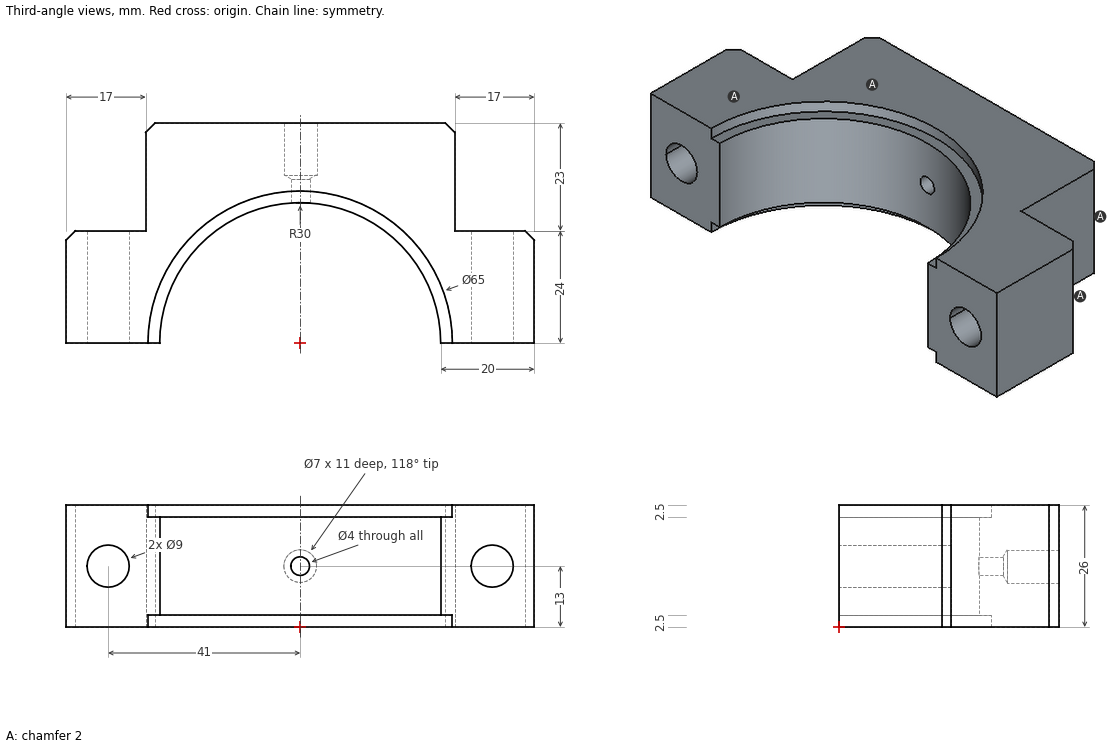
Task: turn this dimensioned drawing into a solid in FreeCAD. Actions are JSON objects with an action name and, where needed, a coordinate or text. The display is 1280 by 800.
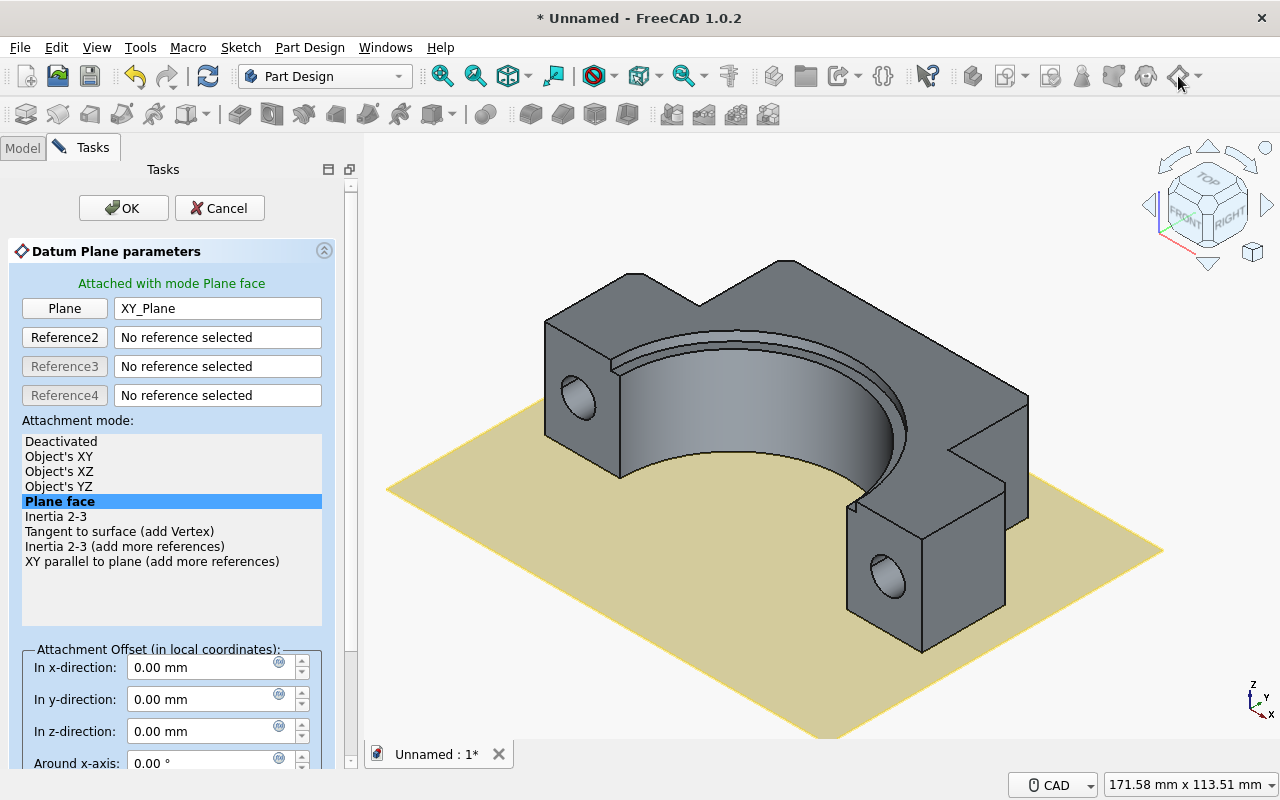
{"action": "triple_click", "coordinate": [210, 731]}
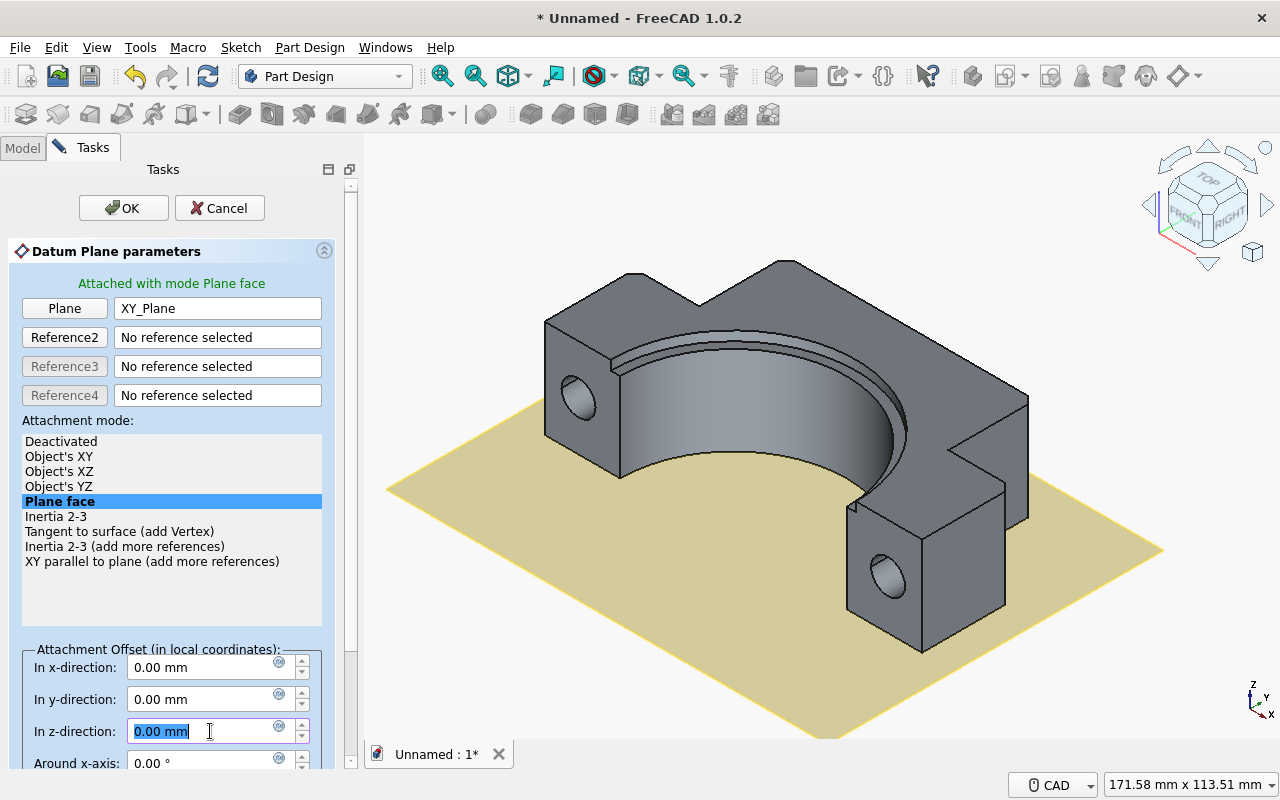
{"action": "type", "text": "2.5"}
{"action": "key", "text": "Tab"}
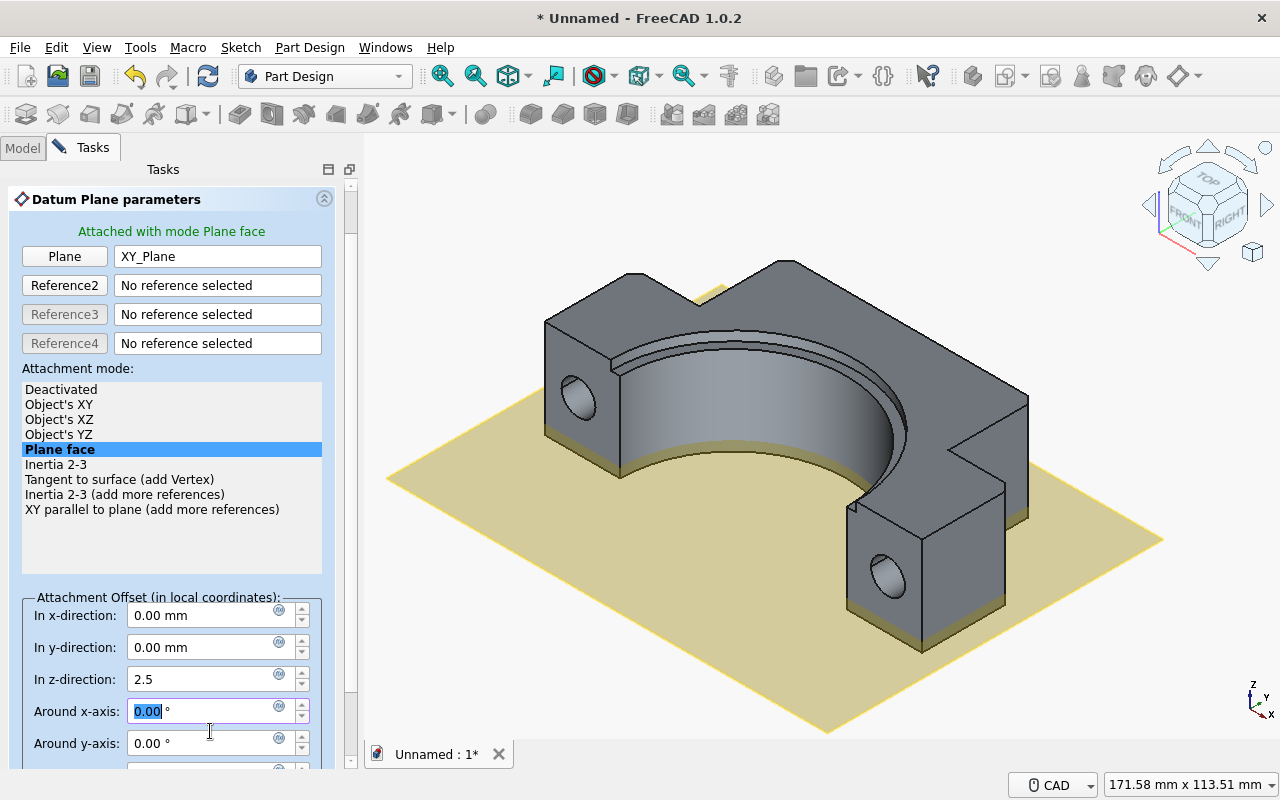
{"action": "scroll", "coordinate": [351, 474], "scroll_direction": "up", "scroll_amount": 2}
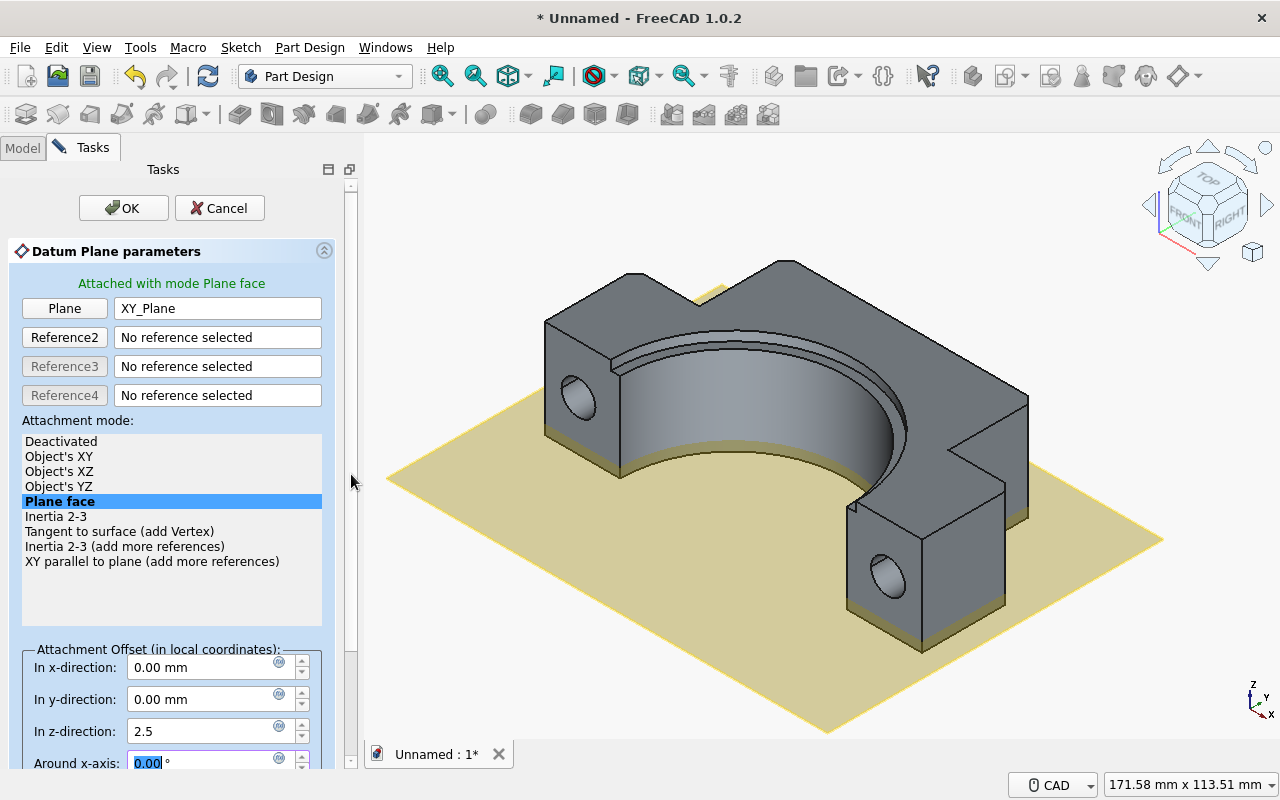
{"action": "left_click", "coordinate": [124, 208]}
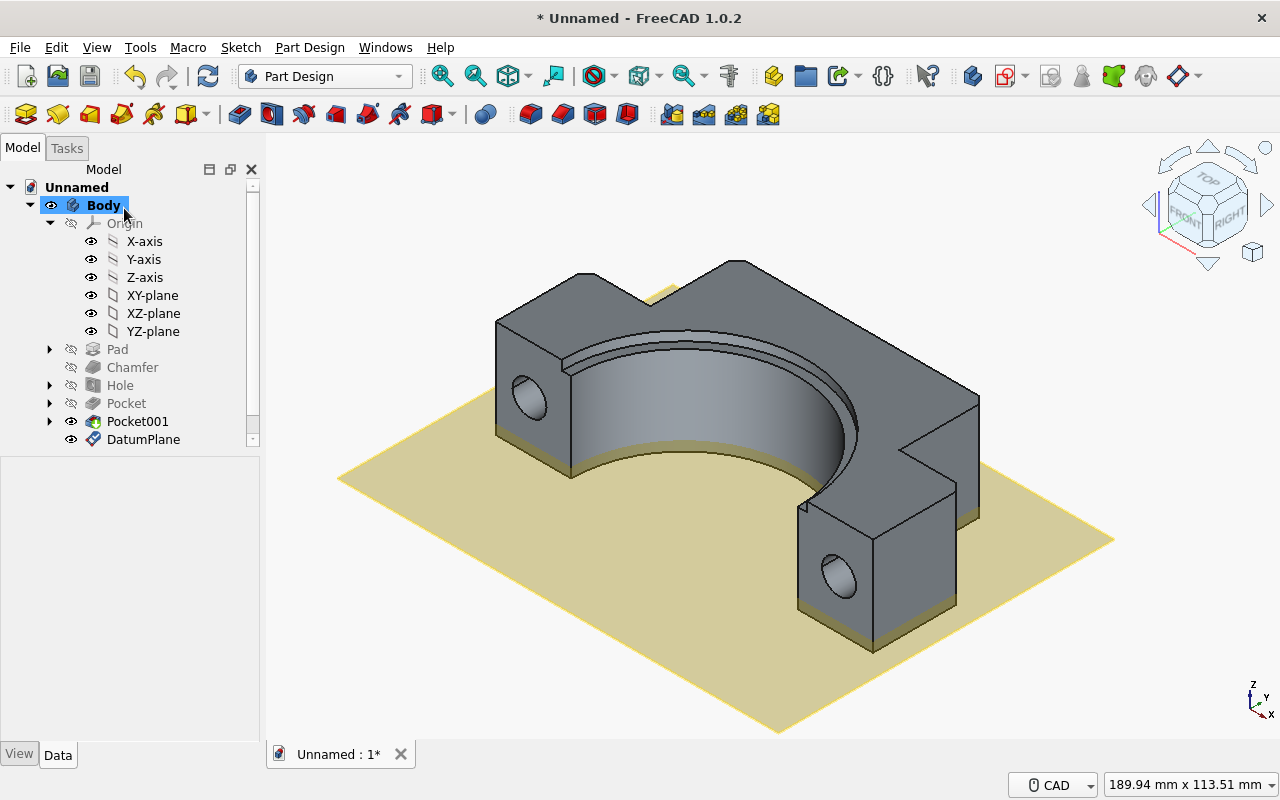
{"action": "left_click", "coordinate": [116, 439]}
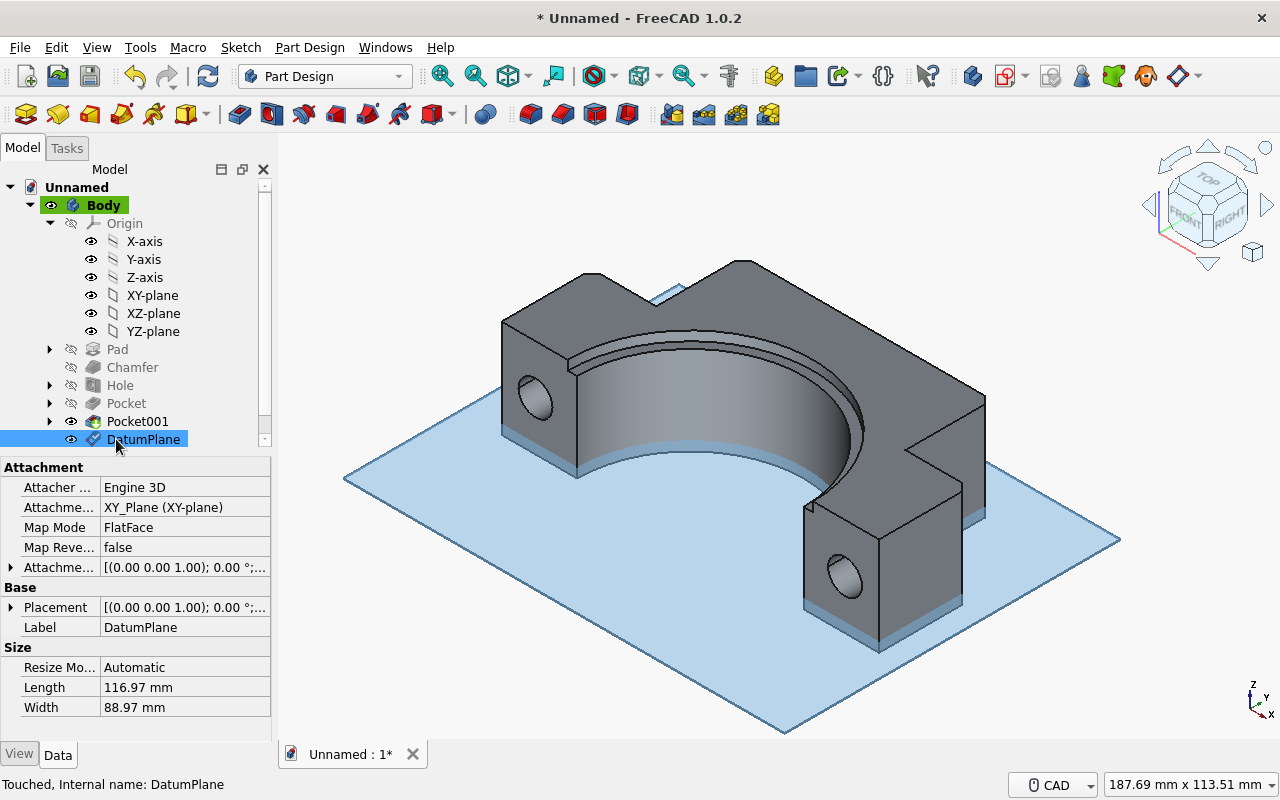
{"action": "left_click", "coordinate": [1006, 76]}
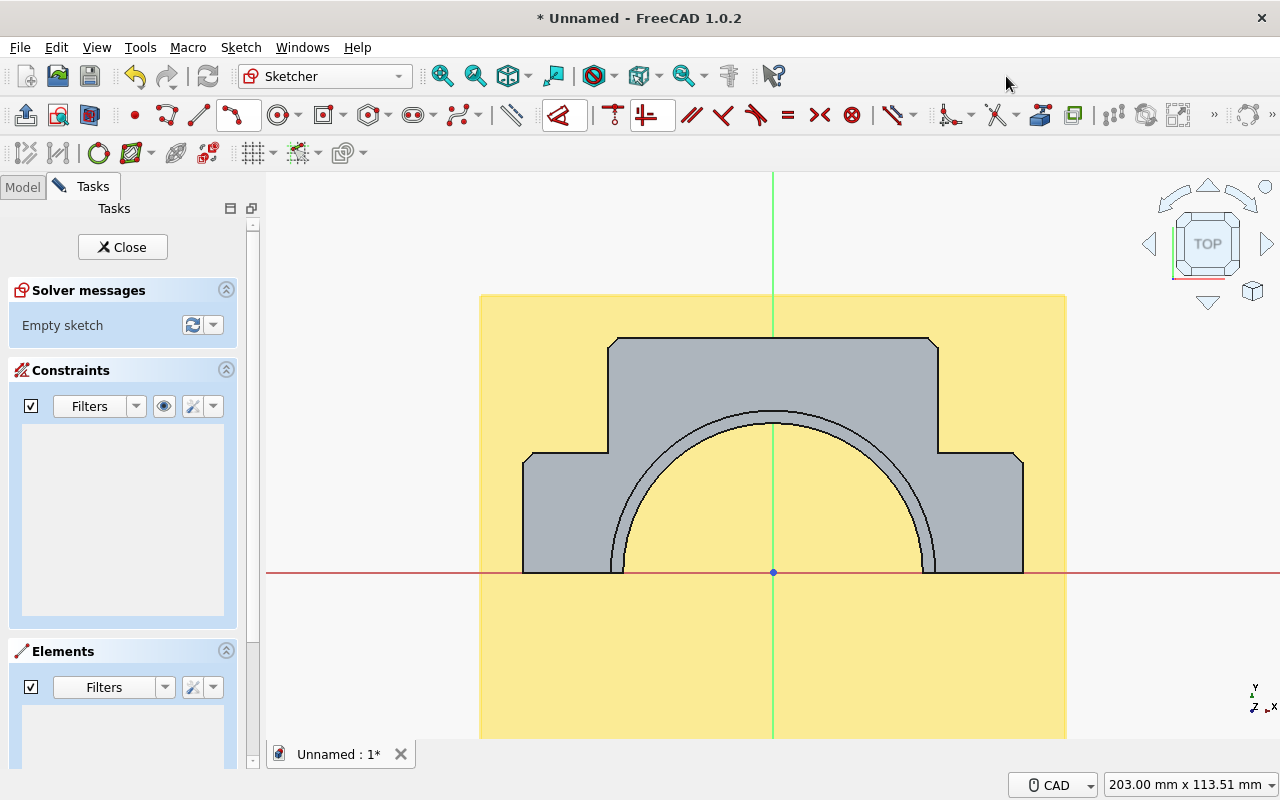
{"action": "key", "text": "q s"}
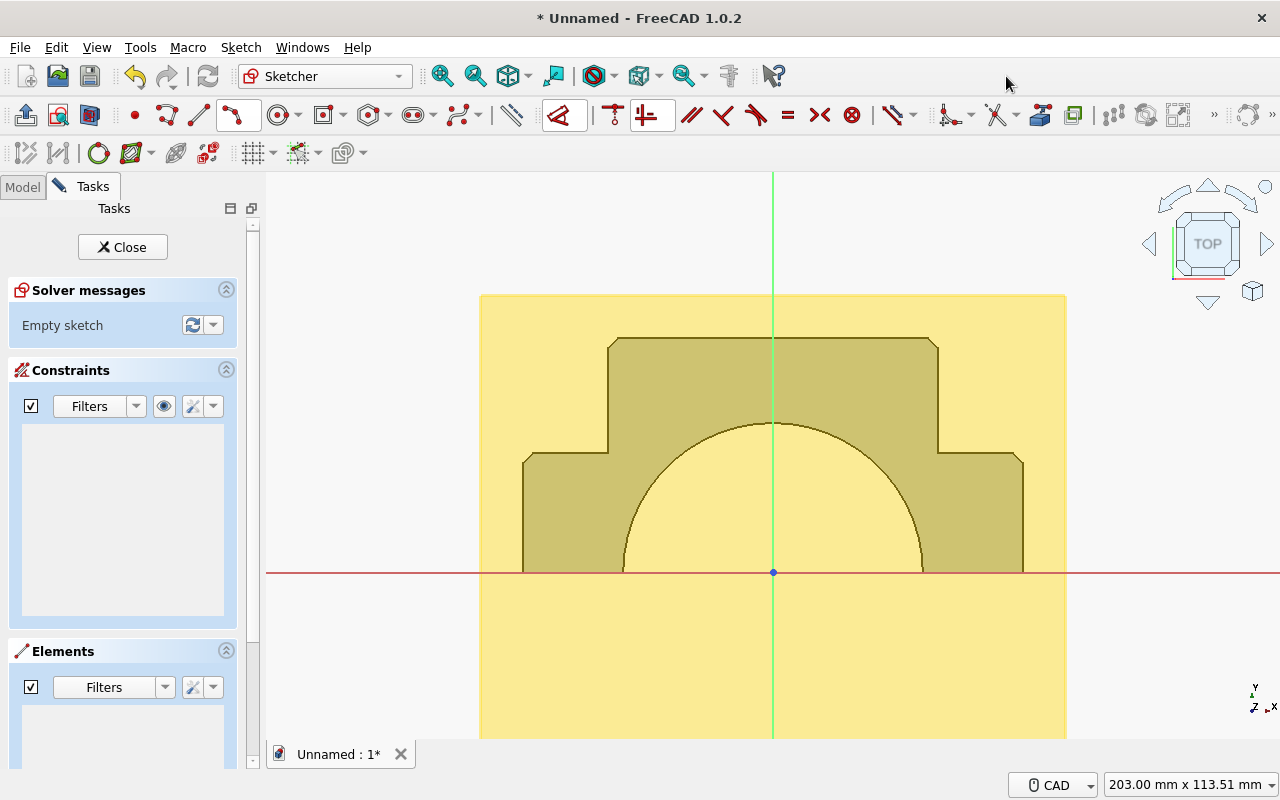
{"action": "scroll", "coordinate": [395, 200], "scroll_direction": "down", "scroll_amount": 1}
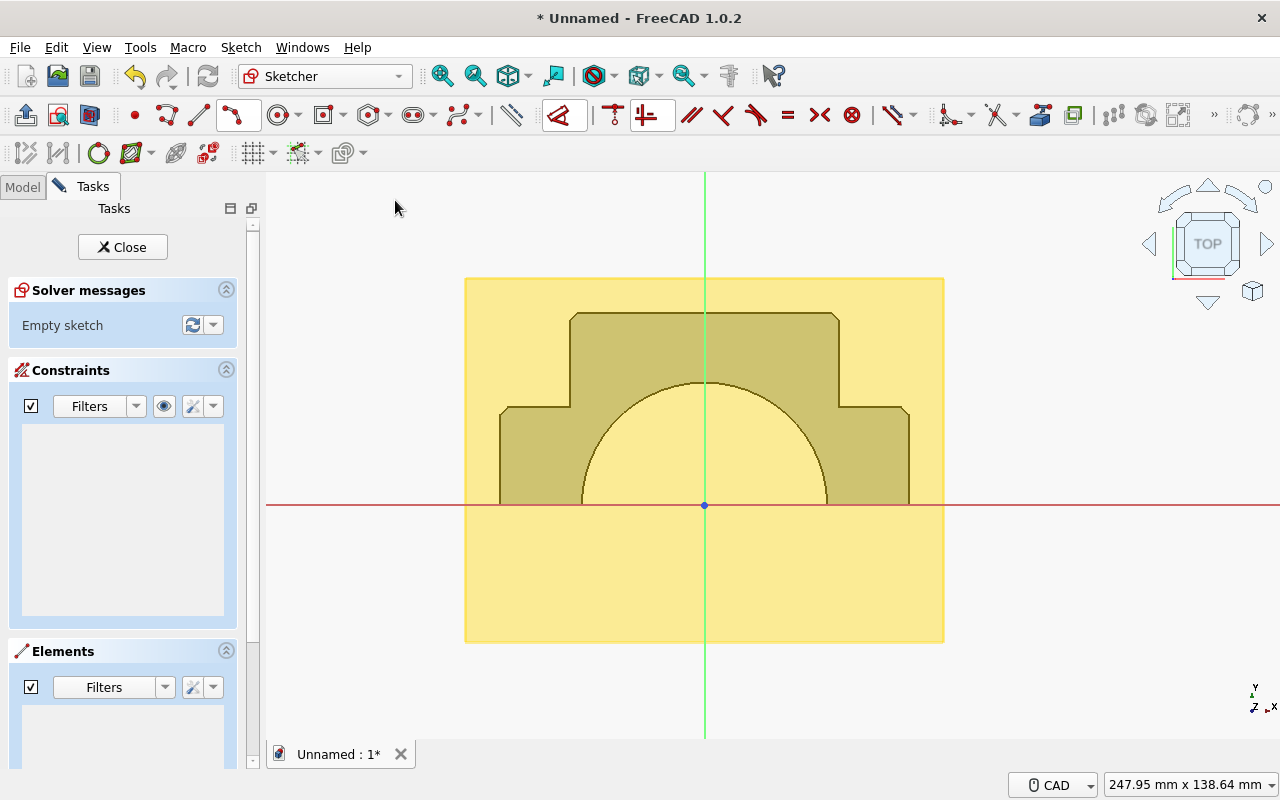
{"action": "scroll", "coordinate": [705, 607], "scroll_direction": "up", "scroll_amount": 2}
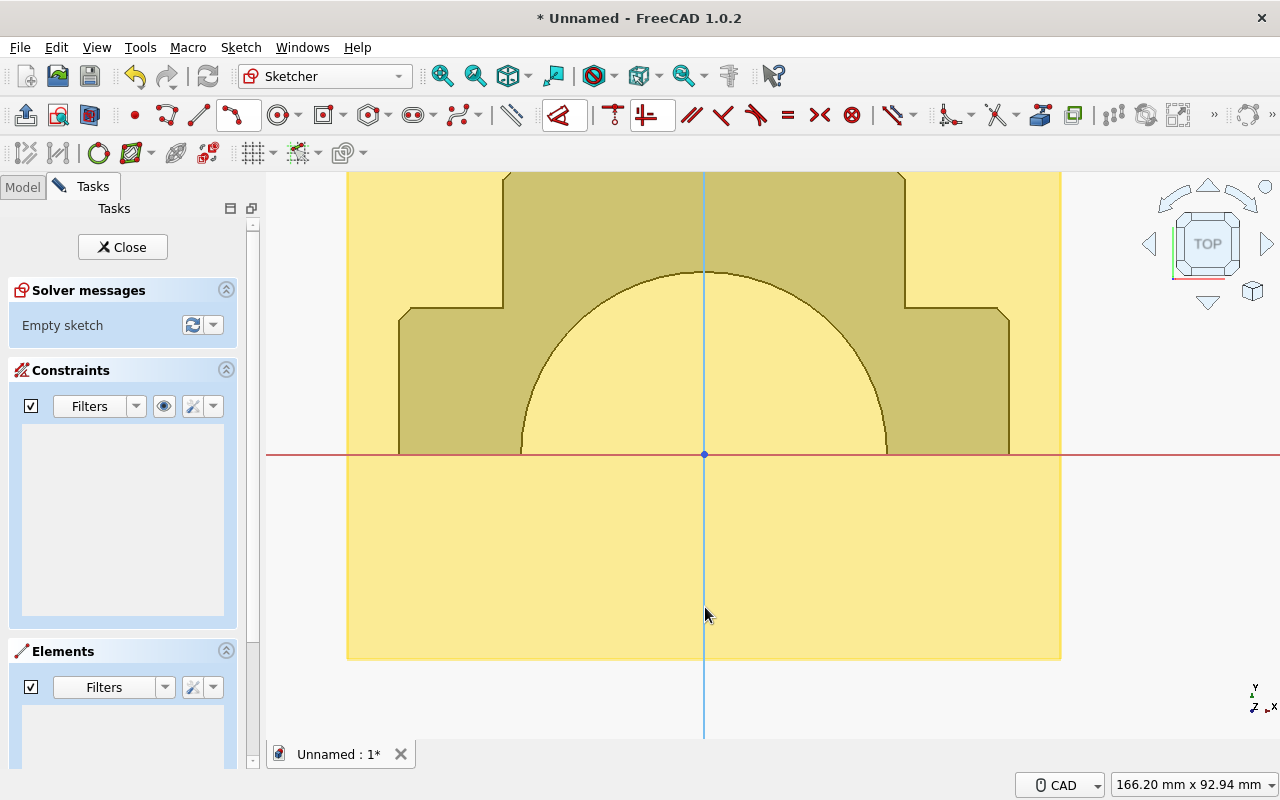
{"action": "key", "text": "g c"}